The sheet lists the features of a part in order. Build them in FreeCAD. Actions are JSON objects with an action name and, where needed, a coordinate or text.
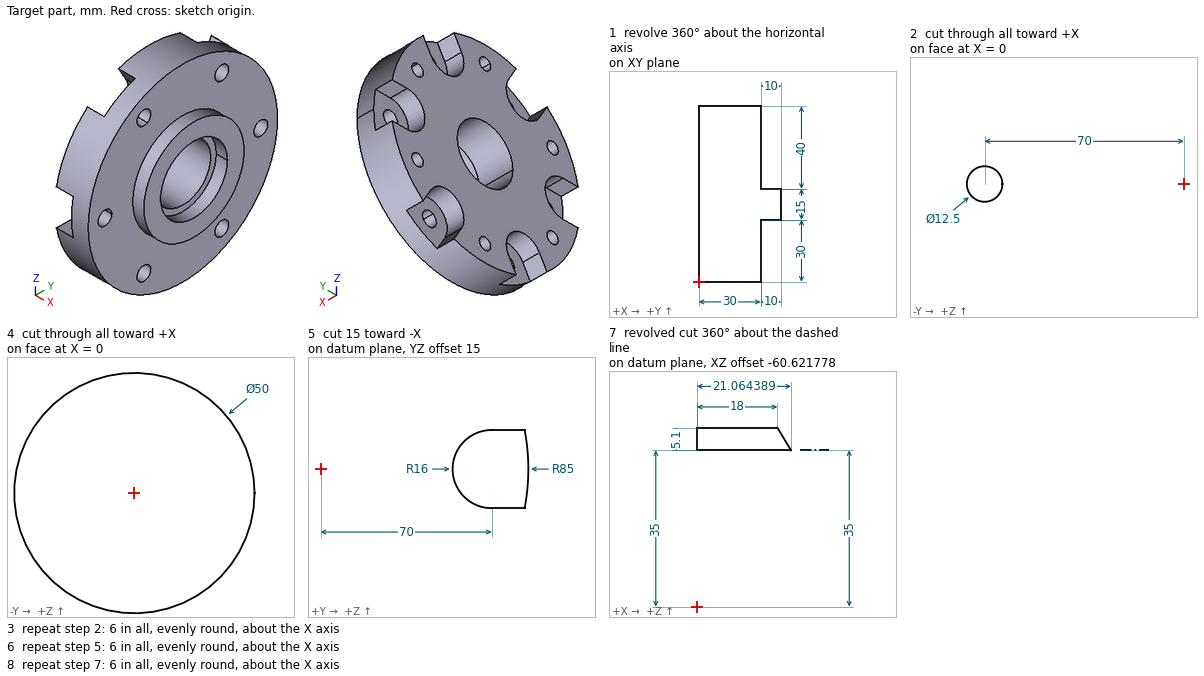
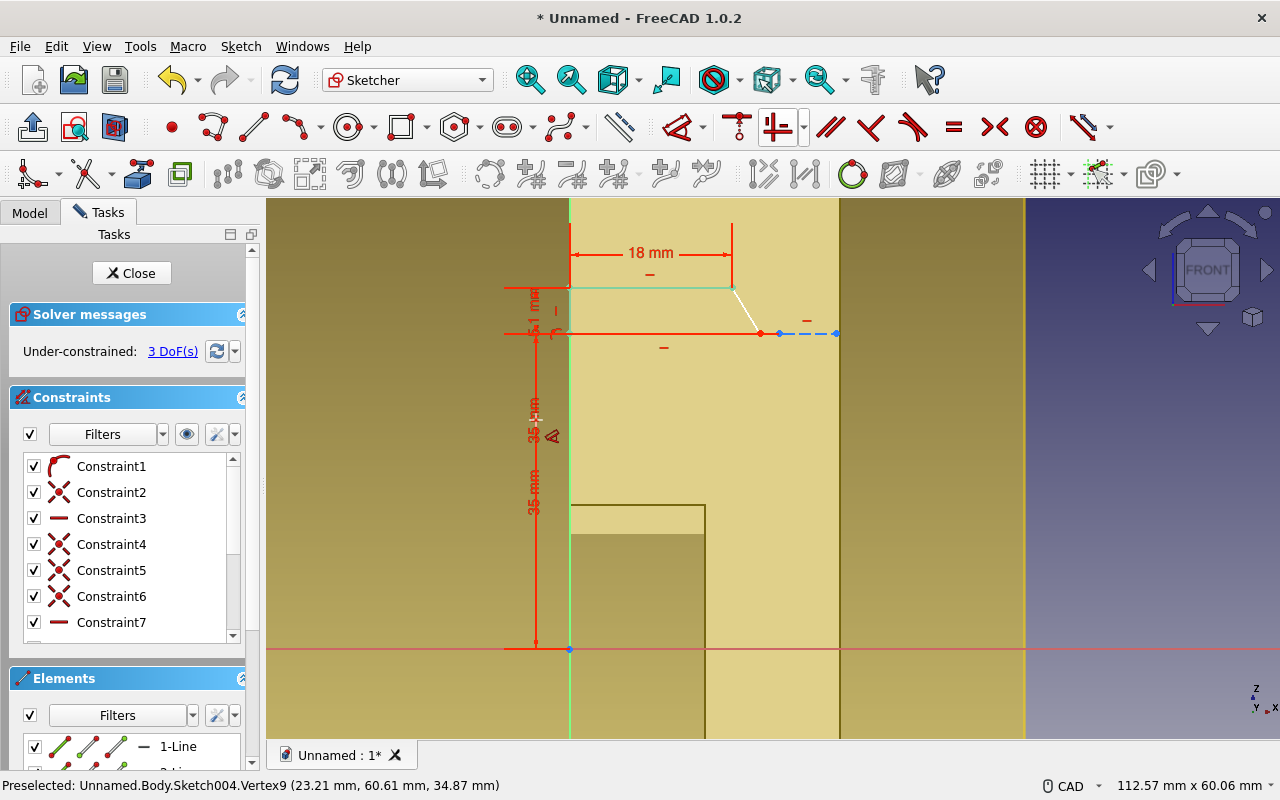
{"action": "left_click", "coordinate": [703, 334]}
{"action": "left_click", "coordinate": [665, 368]}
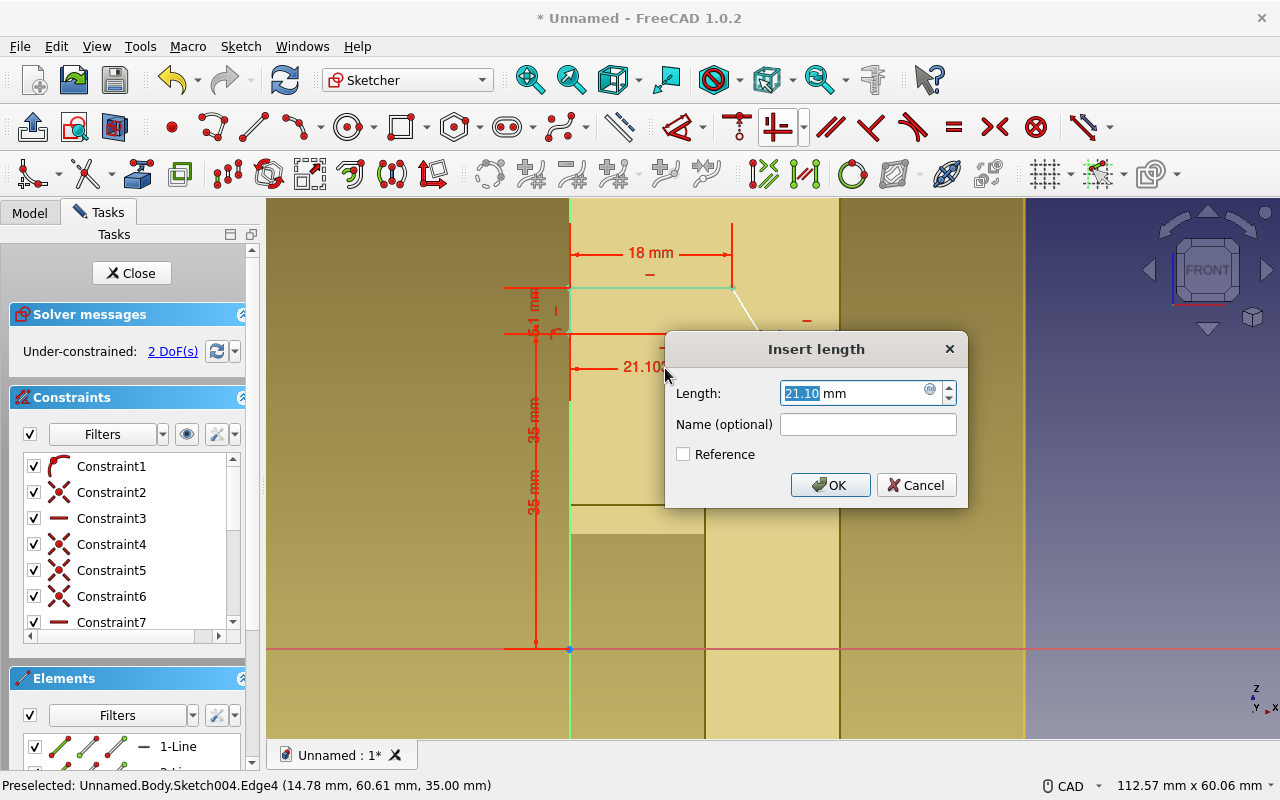
{"action": "type", "text": "21.064389"}
{"action": "key", "text": "Return"}
{"action": "key", "text": "Escape"}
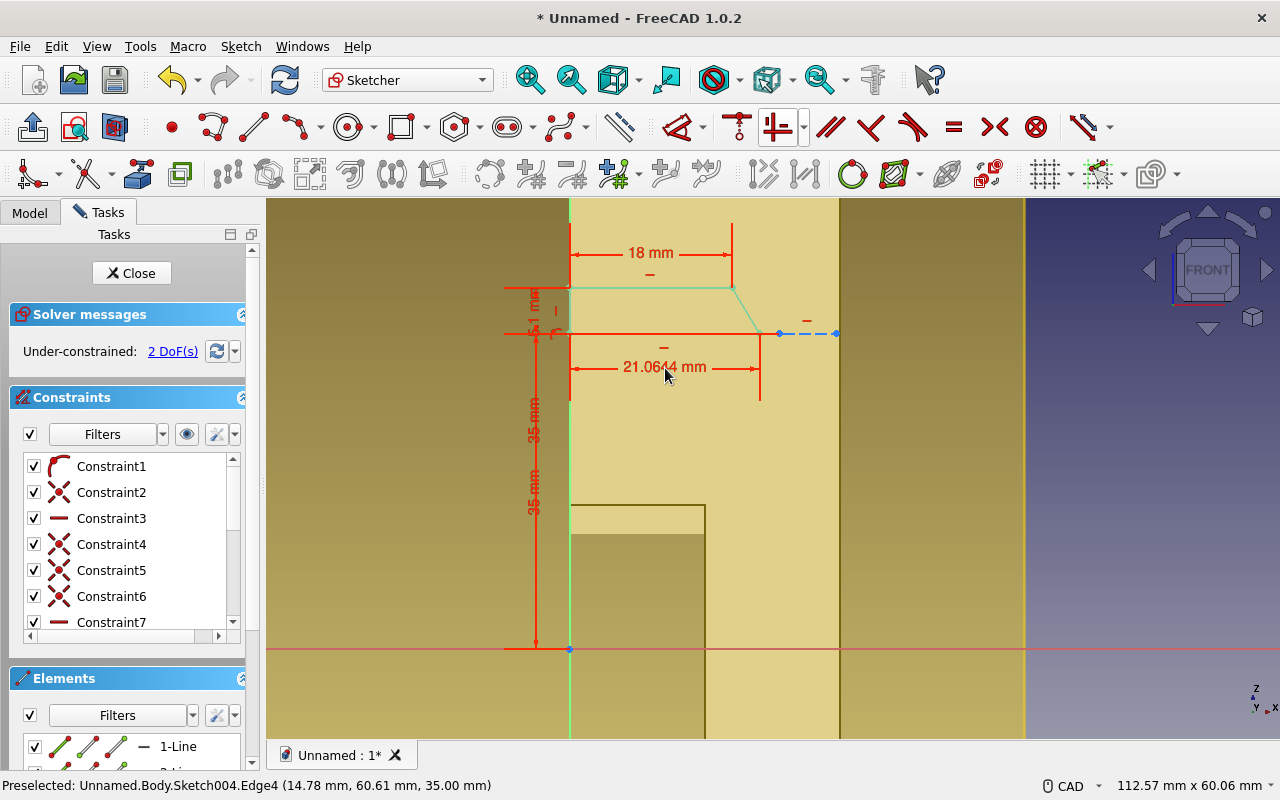
{"action": "left_click", "coordinate": [132, 273]}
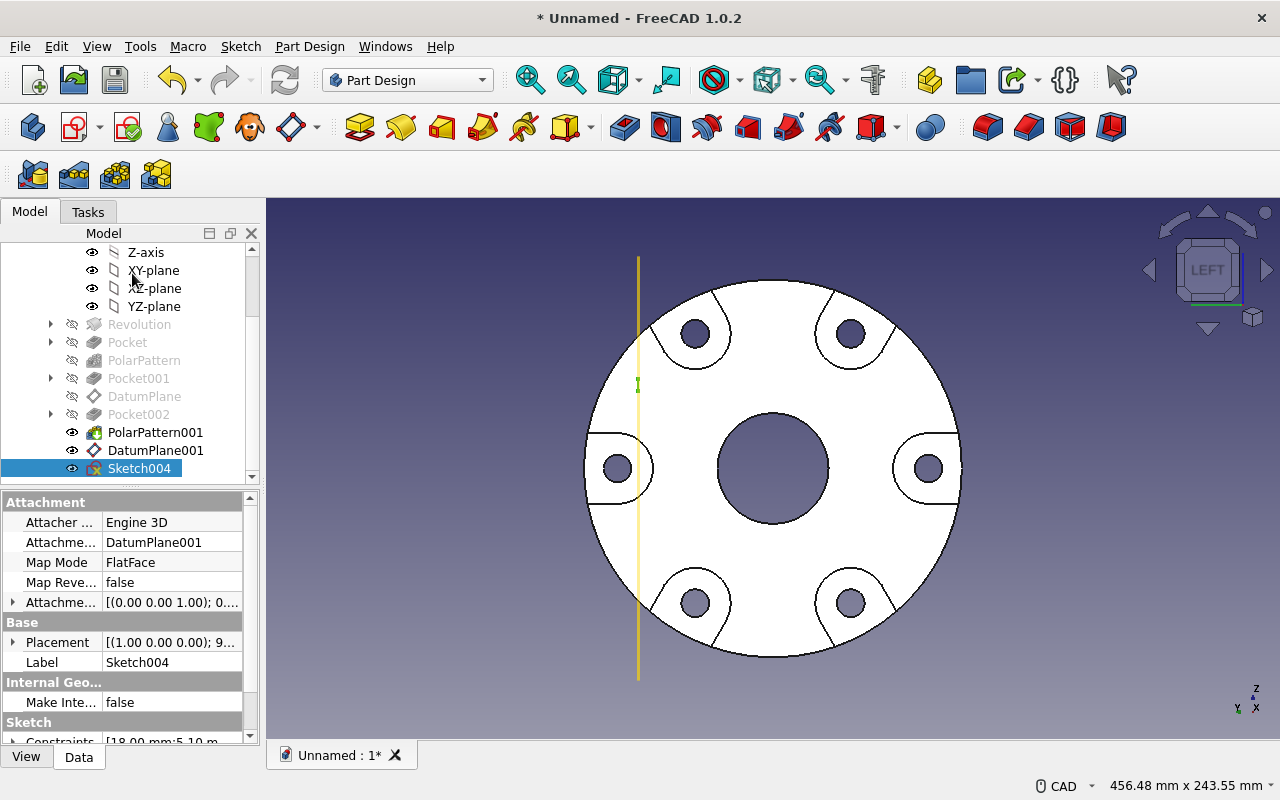
{"action": "left_click", "coordinate": [707, 128]}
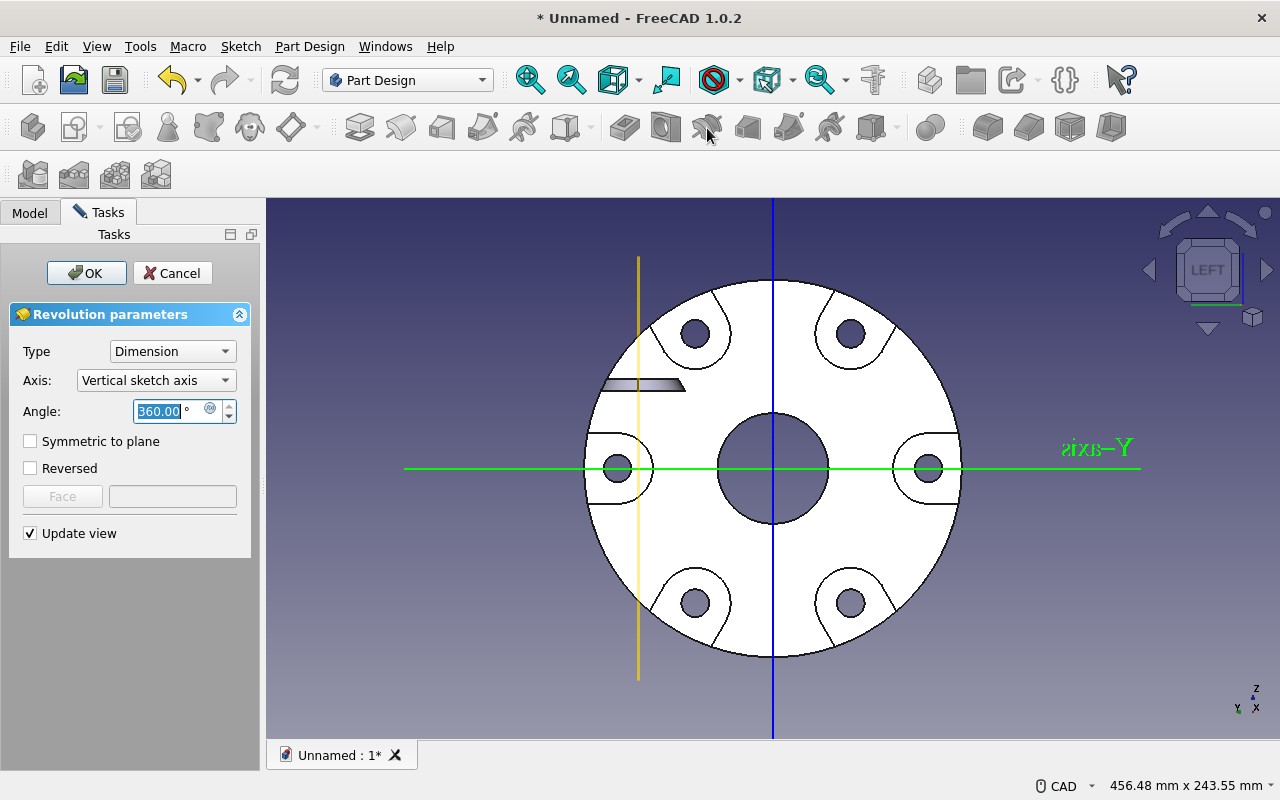
{"action": "left_click", "coordinate": [157, 380]}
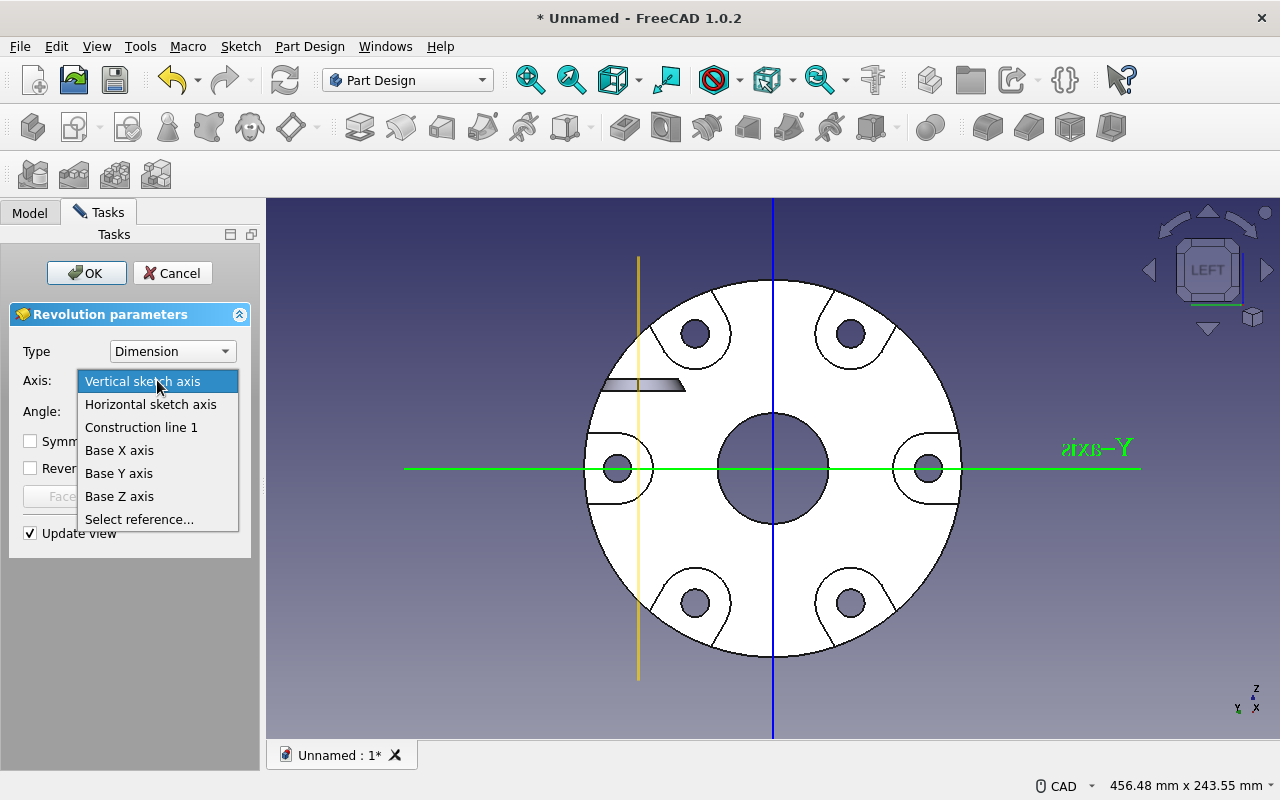
{"action": "left_click", "coordinate": [156, 428]}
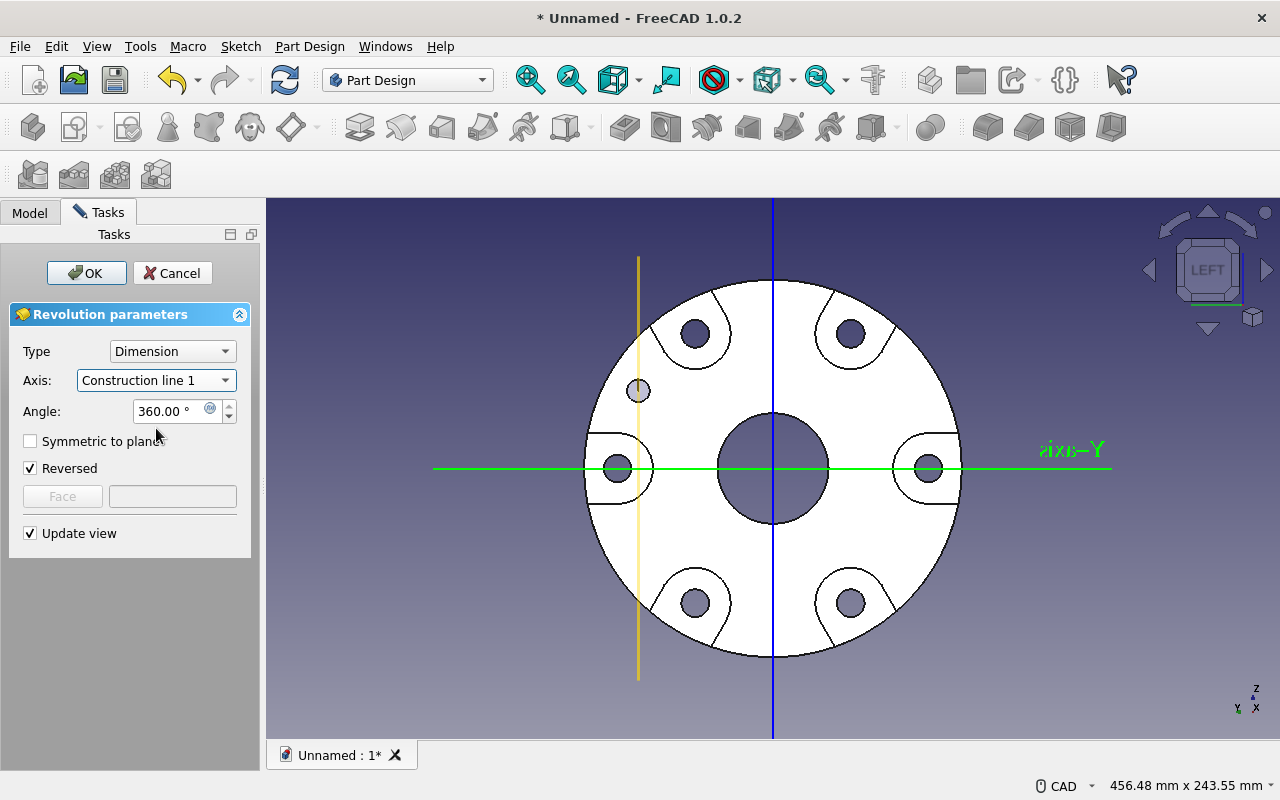
{"action": "left_click", "coordinate": [87, 273]}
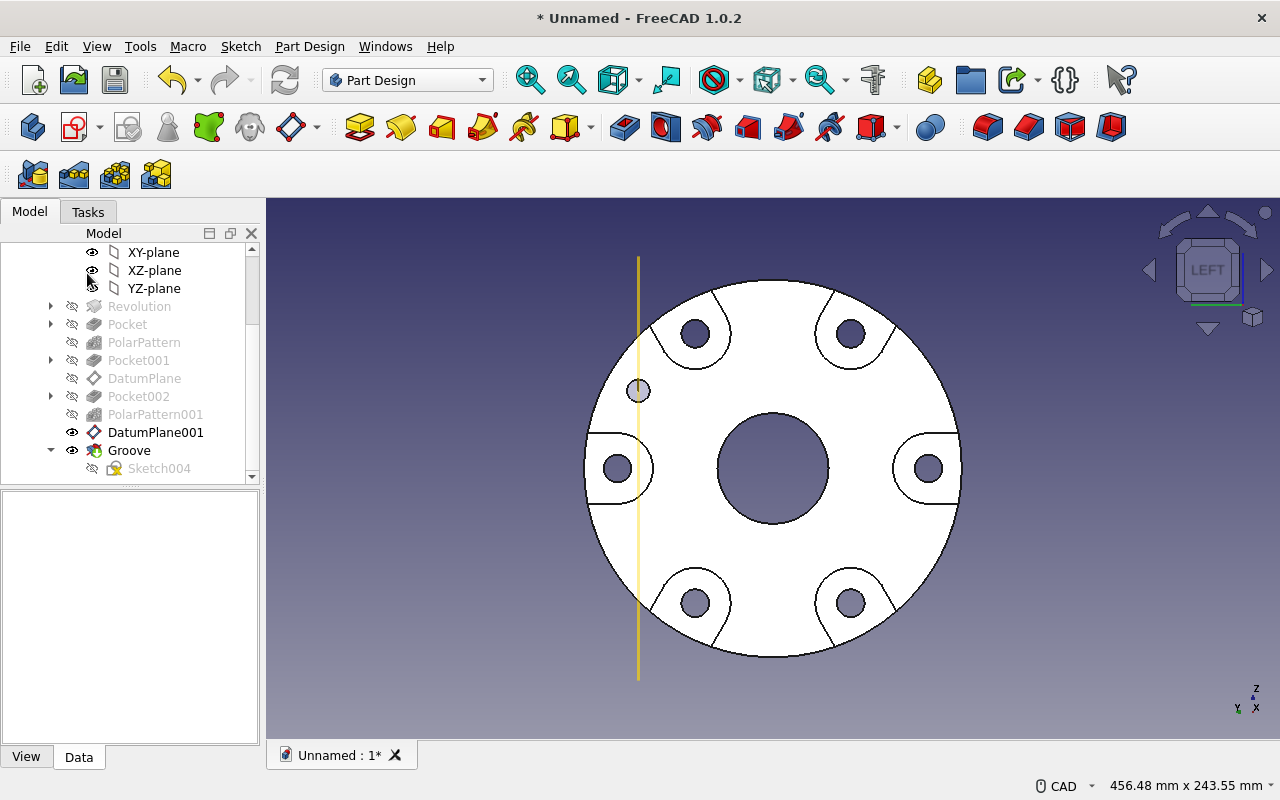
{"action": "left_click", "coordinate": [117, 432]}
{"action": "key", "text": "space"}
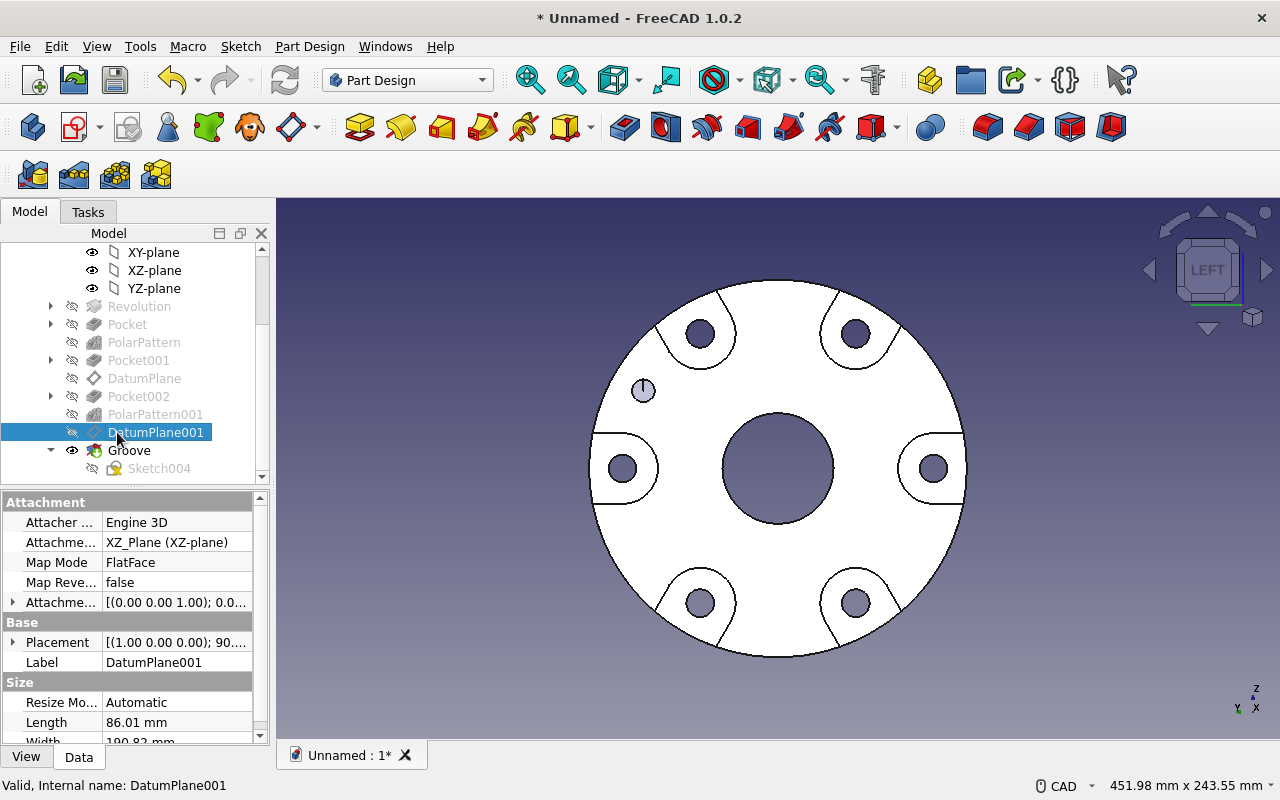
{"action": "left_click", "coordinate": [117, 450]}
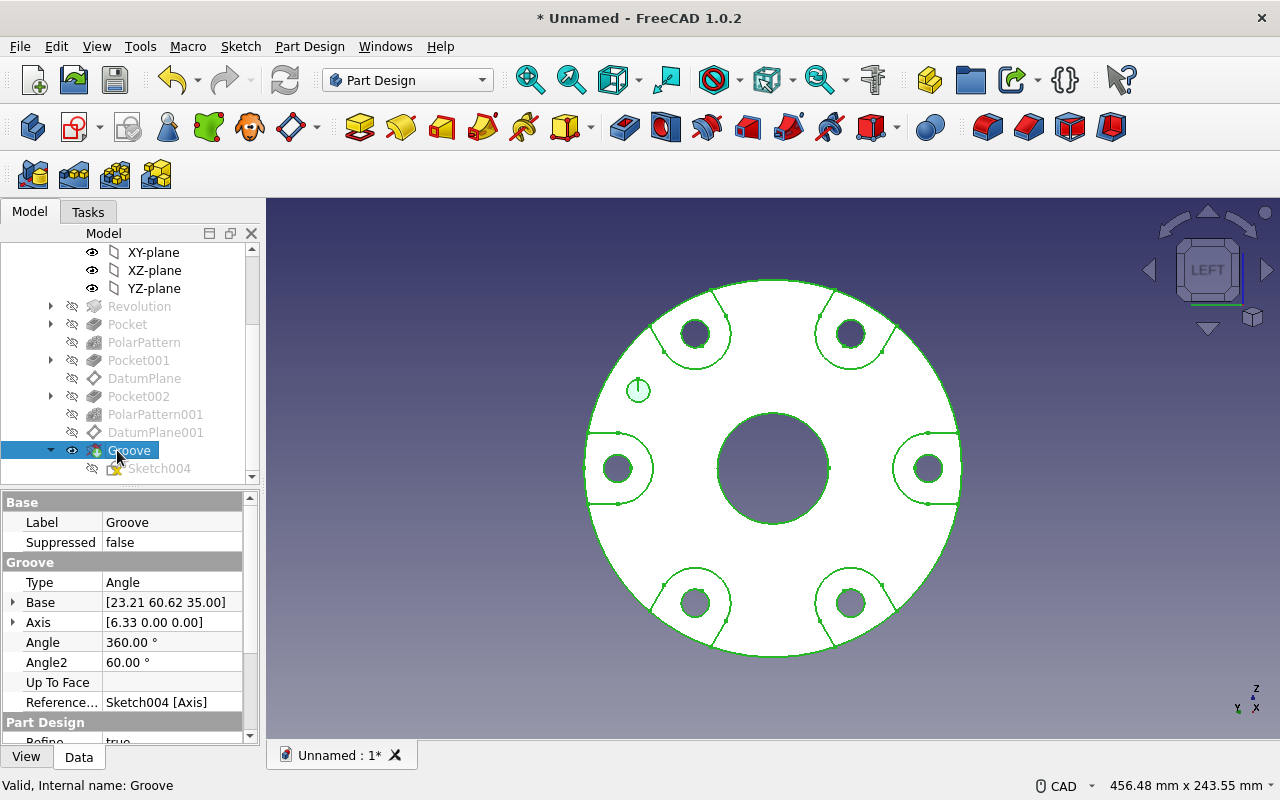
{"action": "left_click", "coordinate": [115, 174]}